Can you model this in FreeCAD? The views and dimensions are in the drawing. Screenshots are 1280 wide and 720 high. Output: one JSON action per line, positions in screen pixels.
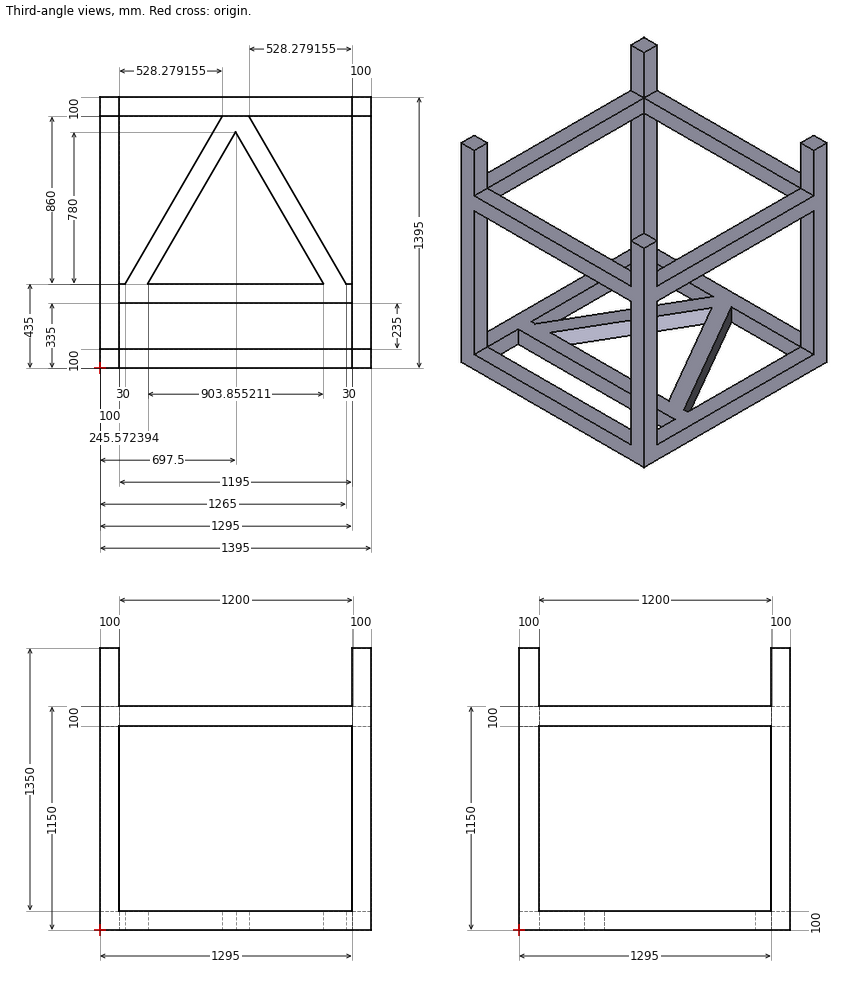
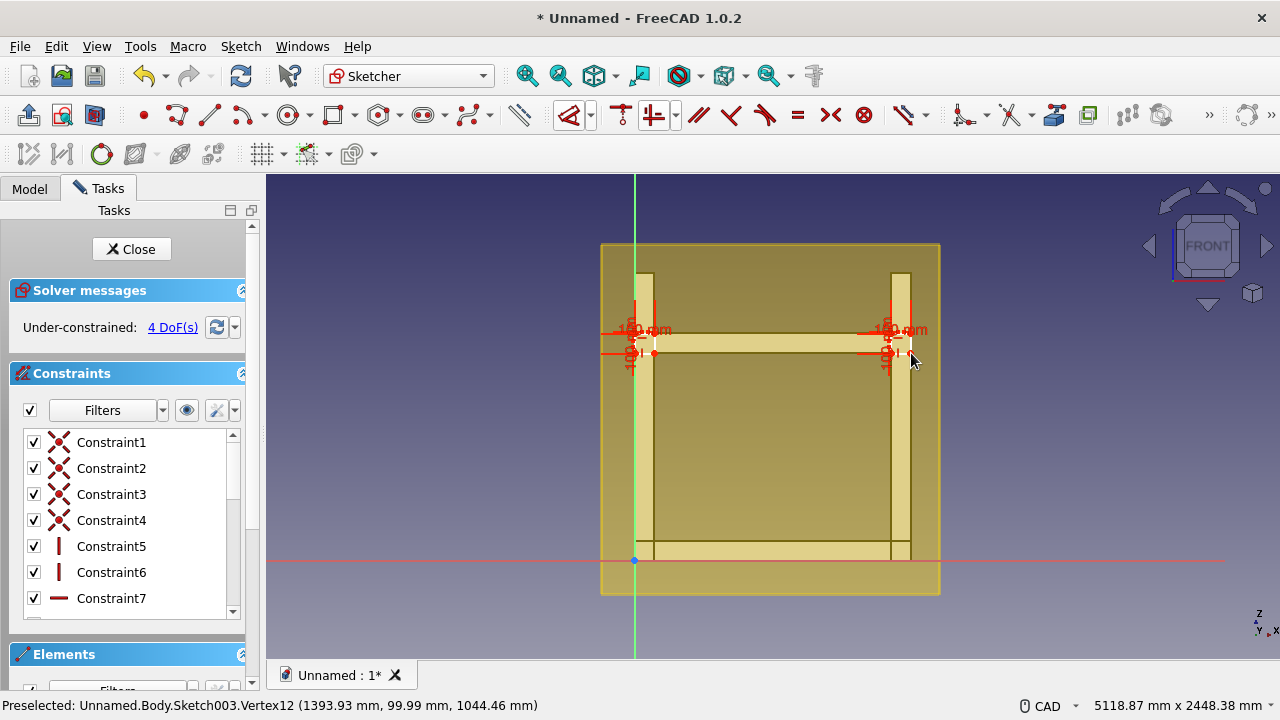
{"action": "left_click", "coordinate": [635, 334]}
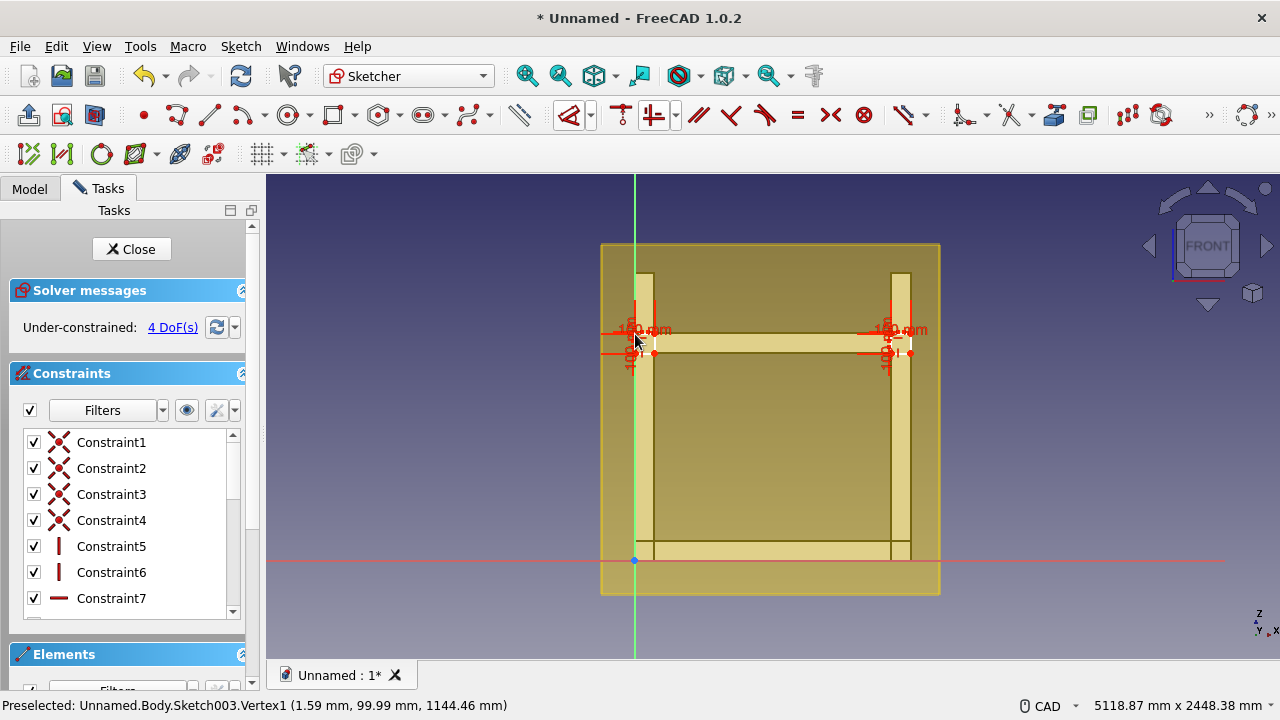
{"action": "left_click", "coordinate": [635, 600]}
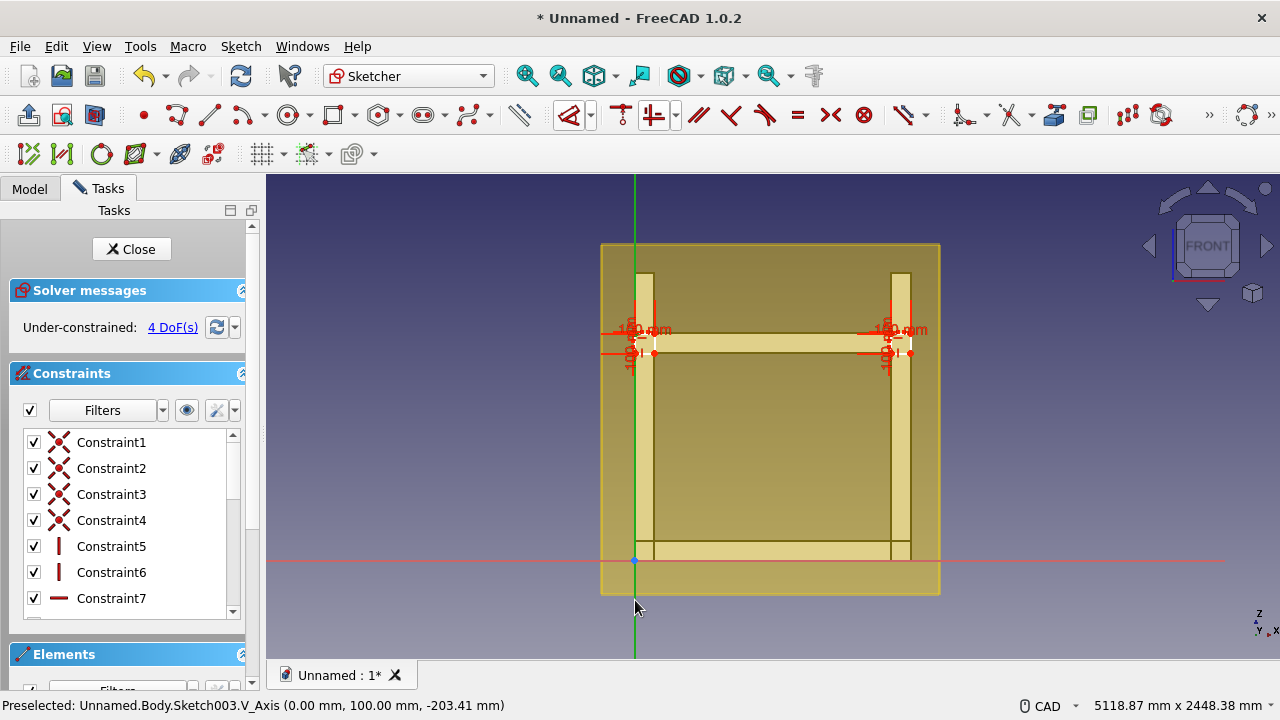
{"action": "left_click", "coordinate": [621, 116]}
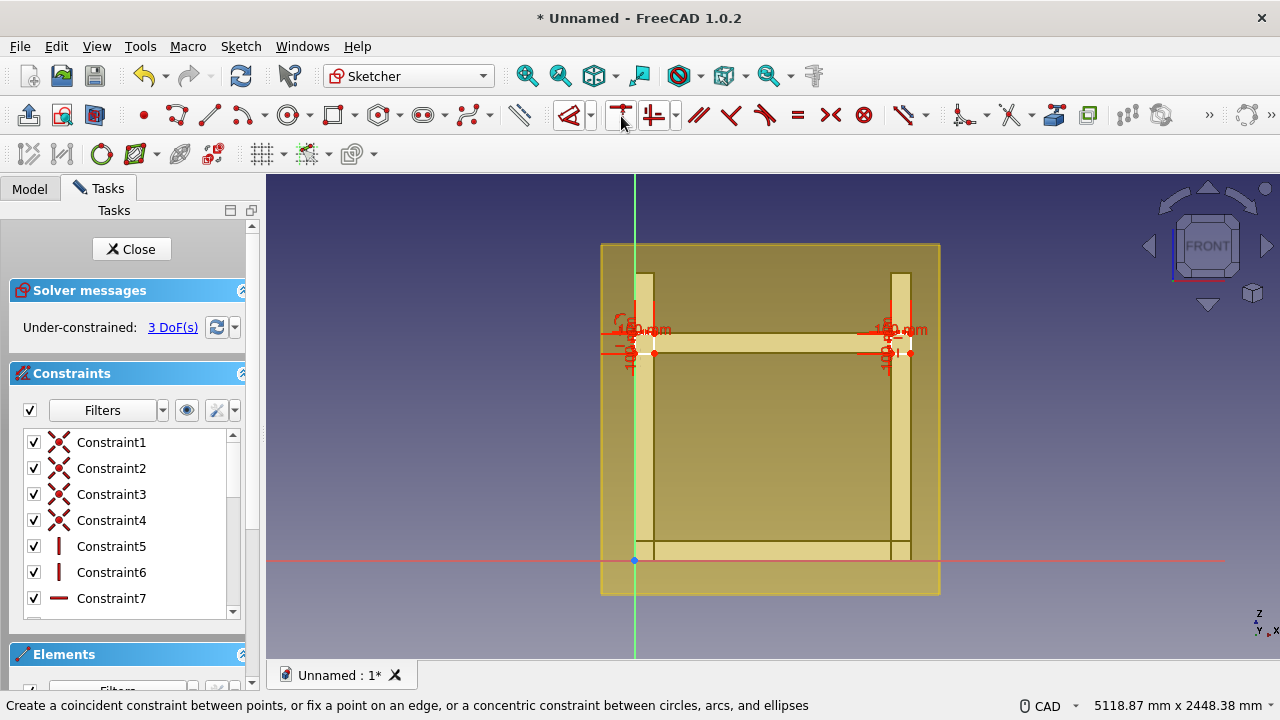
{"action": "left_click", "coordinate": [635, 334]}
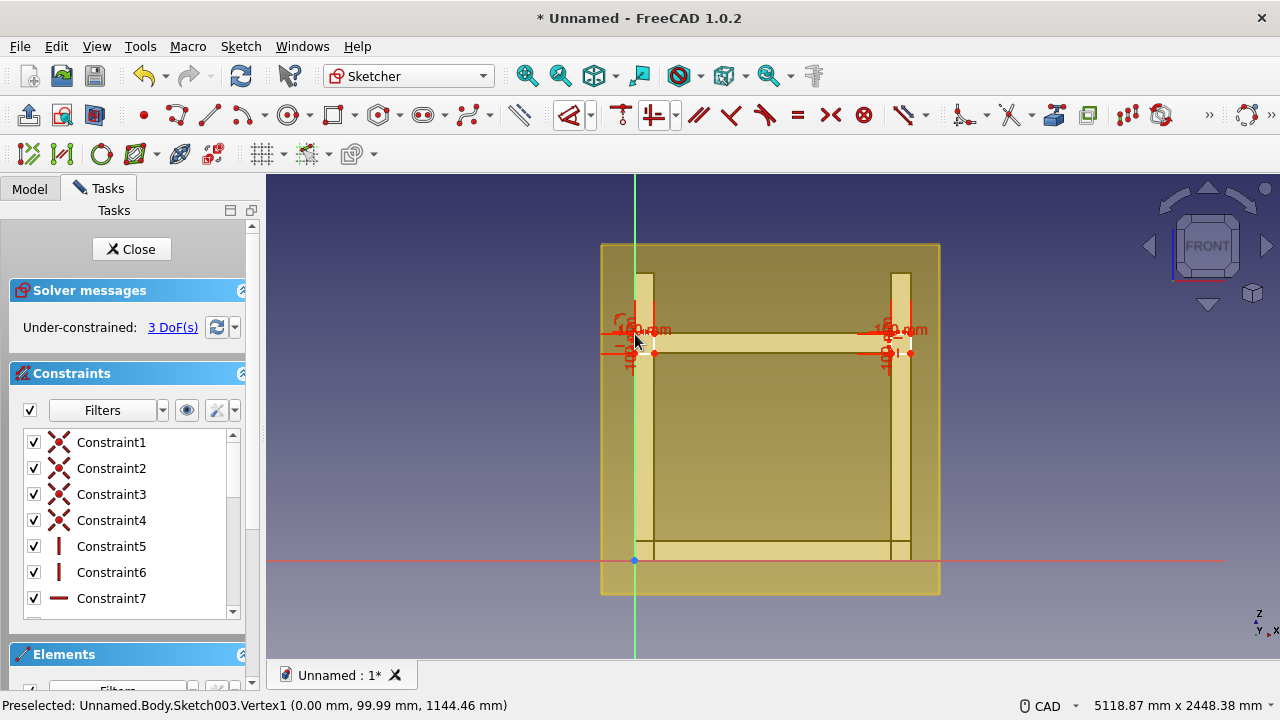
{"action": "left_click", "coordinate": [590, 116]}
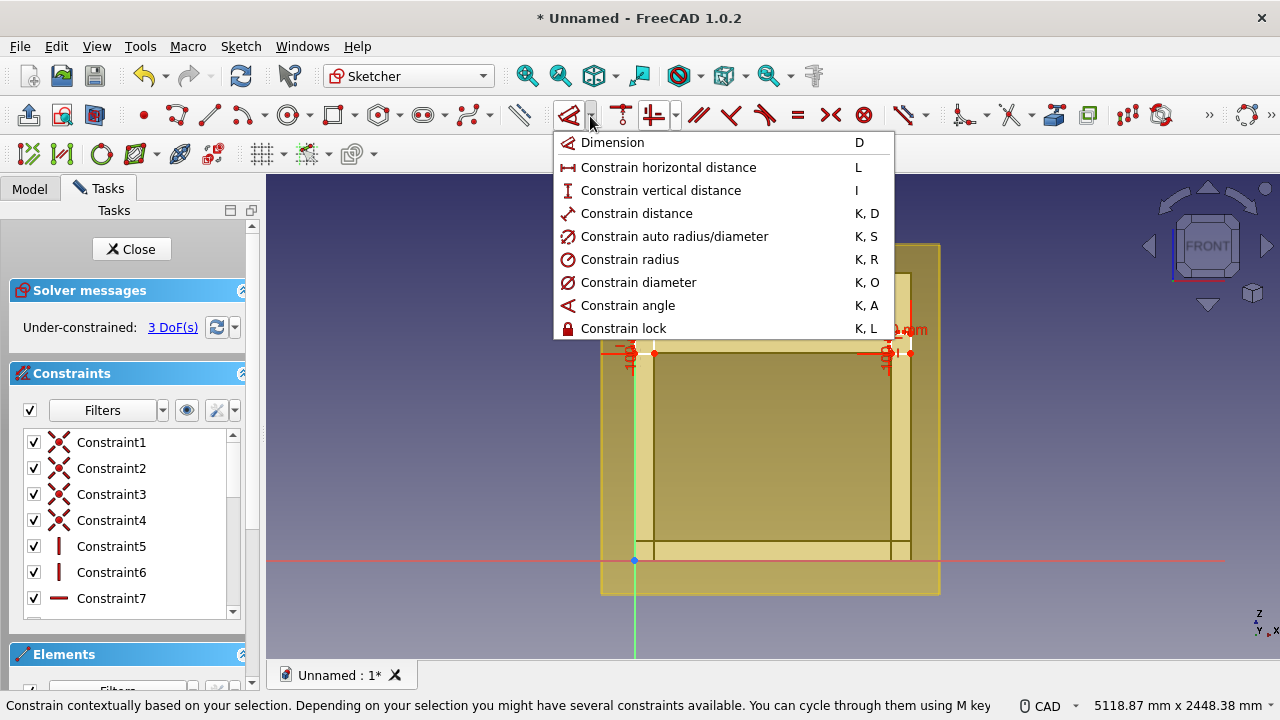
{"action": "left_click", "coordinate": [724, 190]}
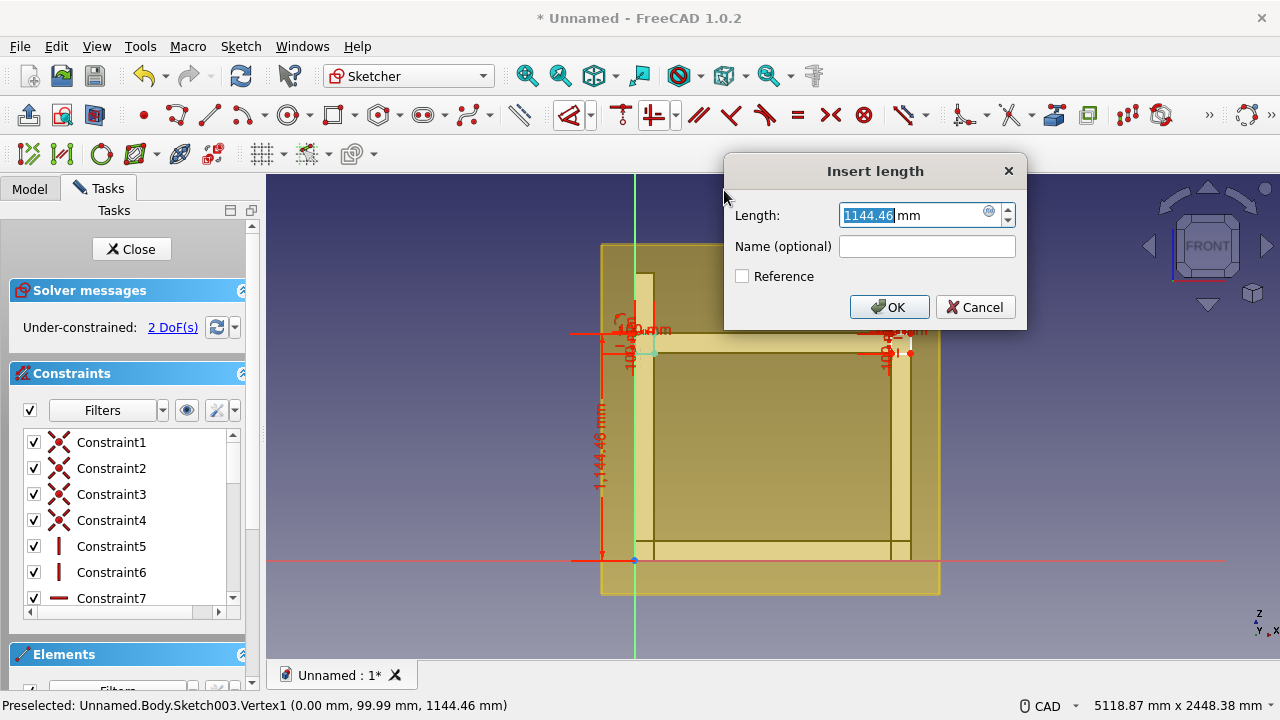
{"action": "type", "text": "1150"}
{"action": "key", "text": "Return"}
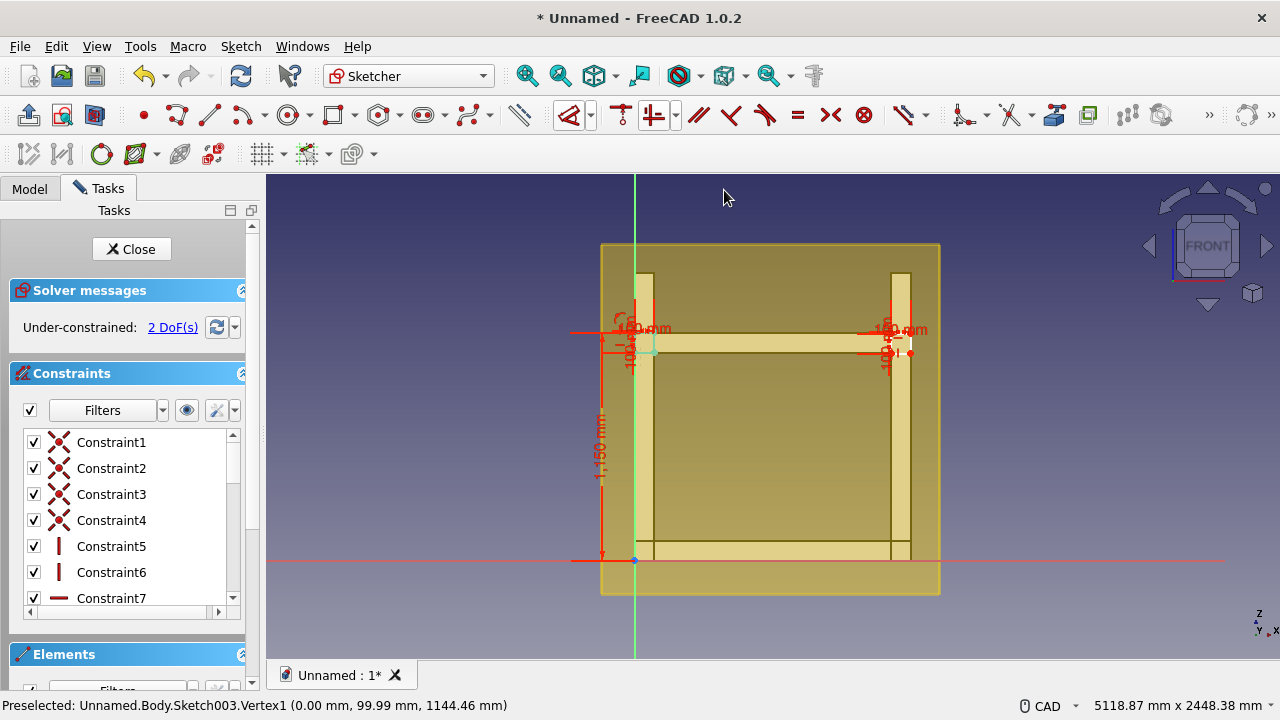
{"action": "left_click", "coordinate": [891, 334]}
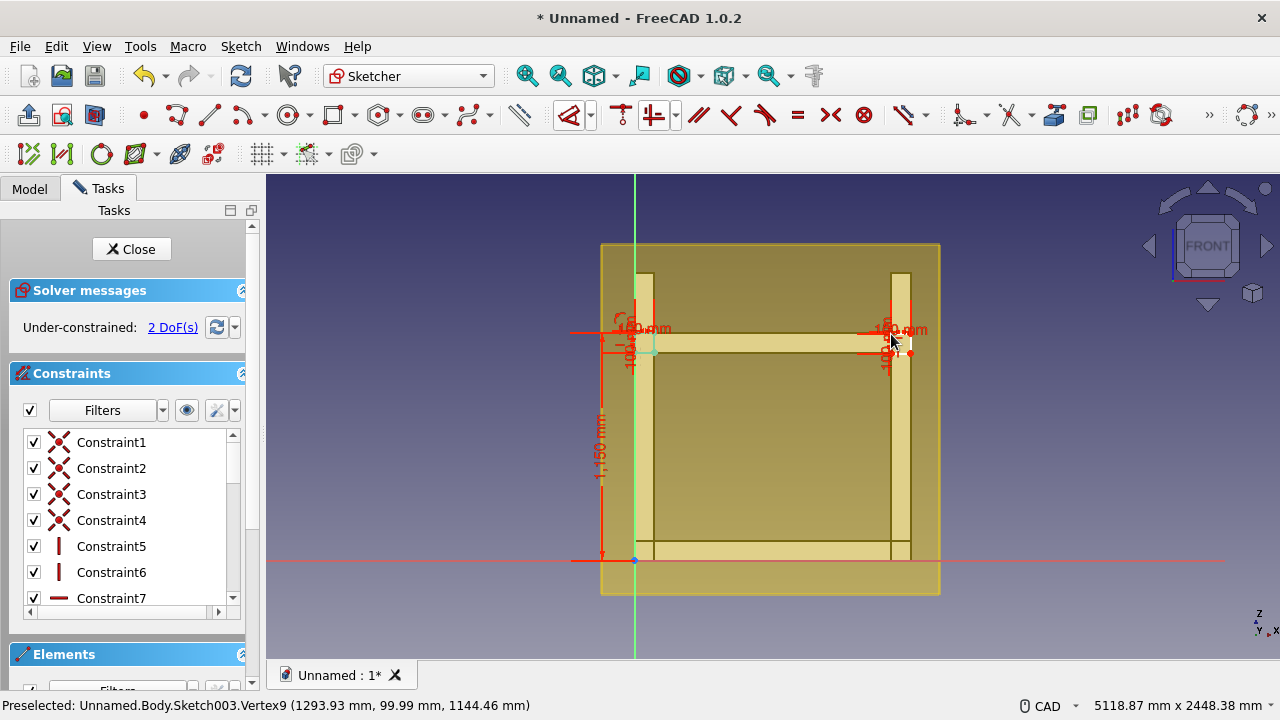
{"action": "left_click", "coordinate": [590, 116]}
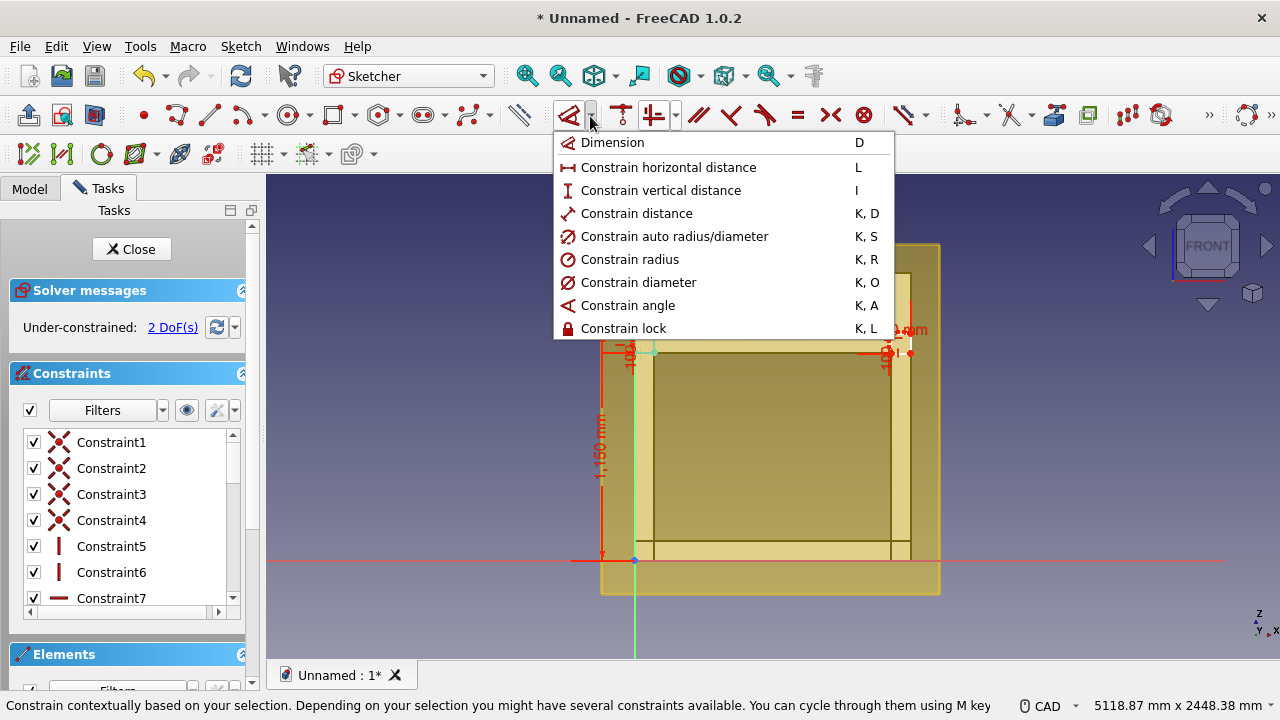
{"action": "left_click", "coordinate": [724, 168]}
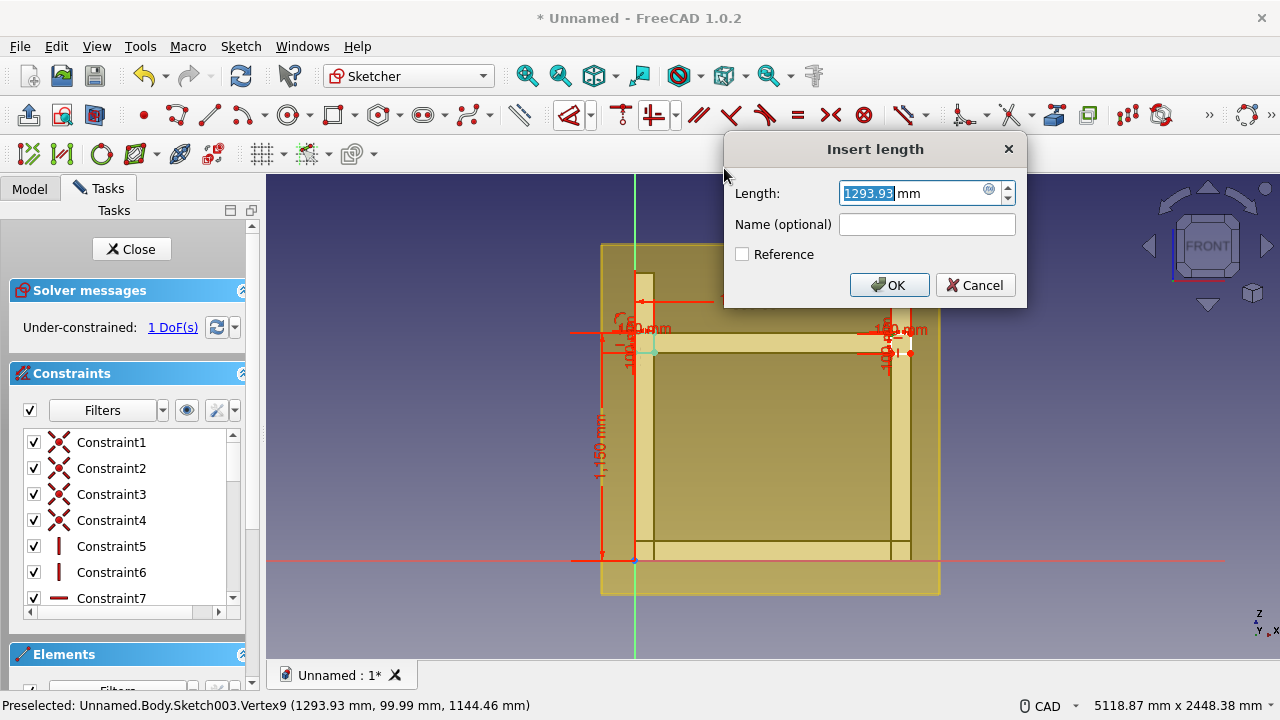
{"action": "type", "text": "1295"}
{"action": "key", "text": "Return"}